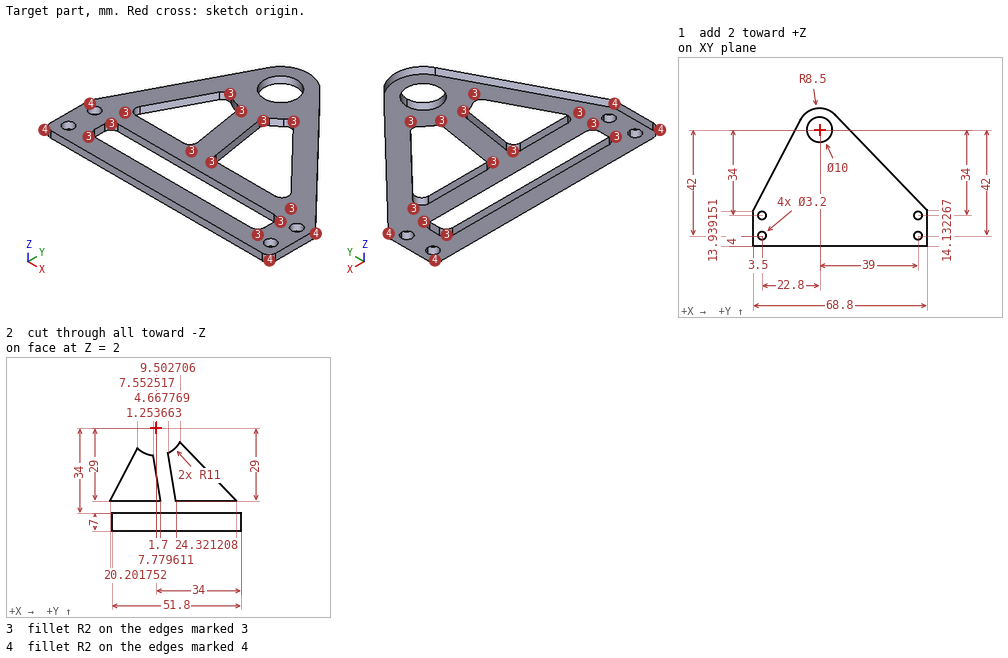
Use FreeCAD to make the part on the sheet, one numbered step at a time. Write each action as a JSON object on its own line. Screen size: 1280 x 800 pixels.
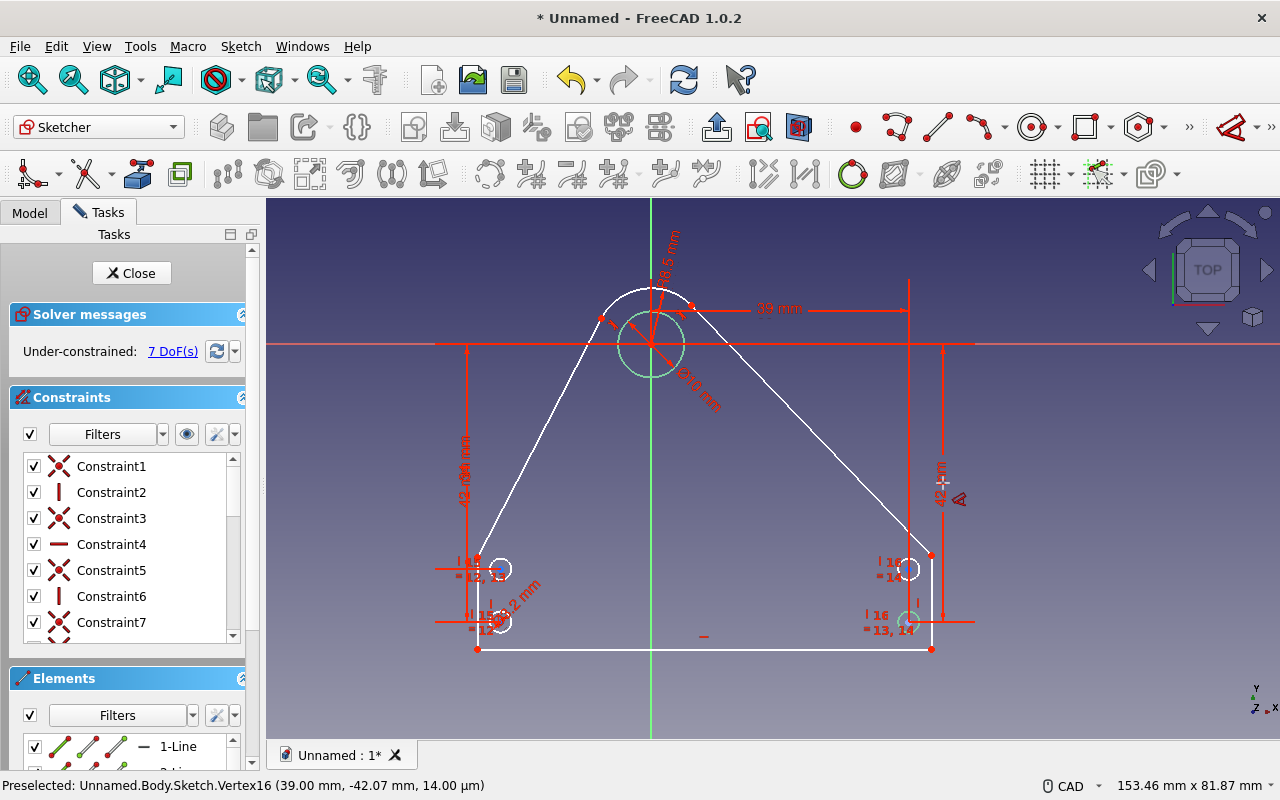
{"action": "left_click", "coordinate": [909, 569]}
{"action": "left_click", "coordinate": [943, 457]}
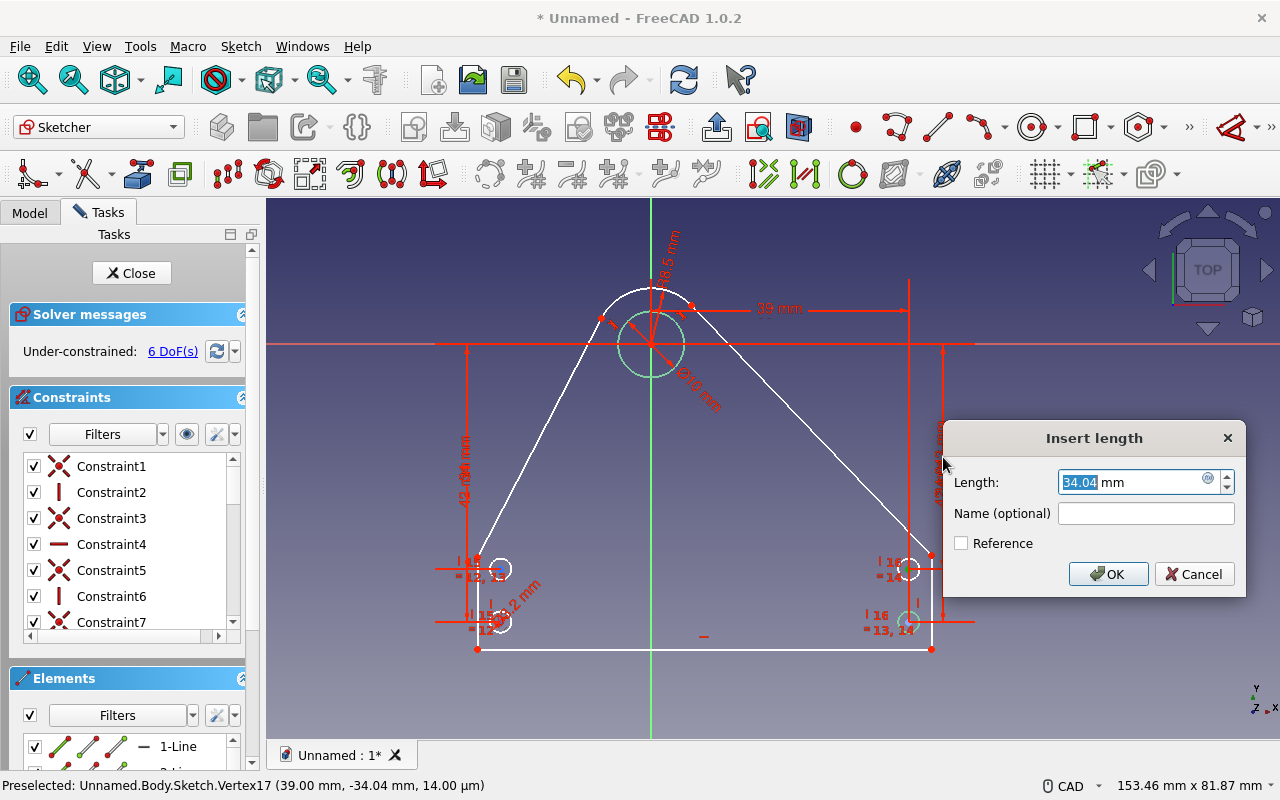
{"action": "type", "text": "34"}
{"action": "key", "text": "Return"}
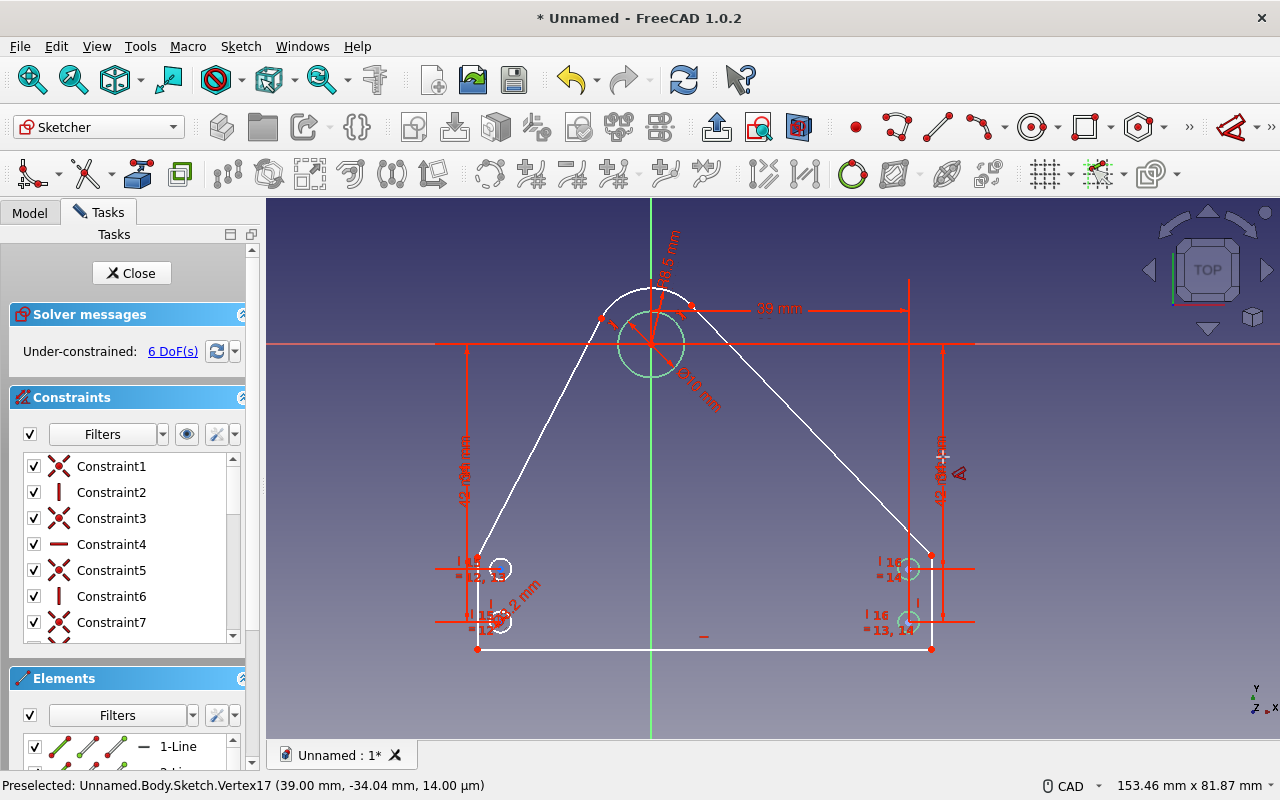
{"action": "scroll", "coordinate": [478, 650], "scroll_direction": "up", "scroll_amount": 3}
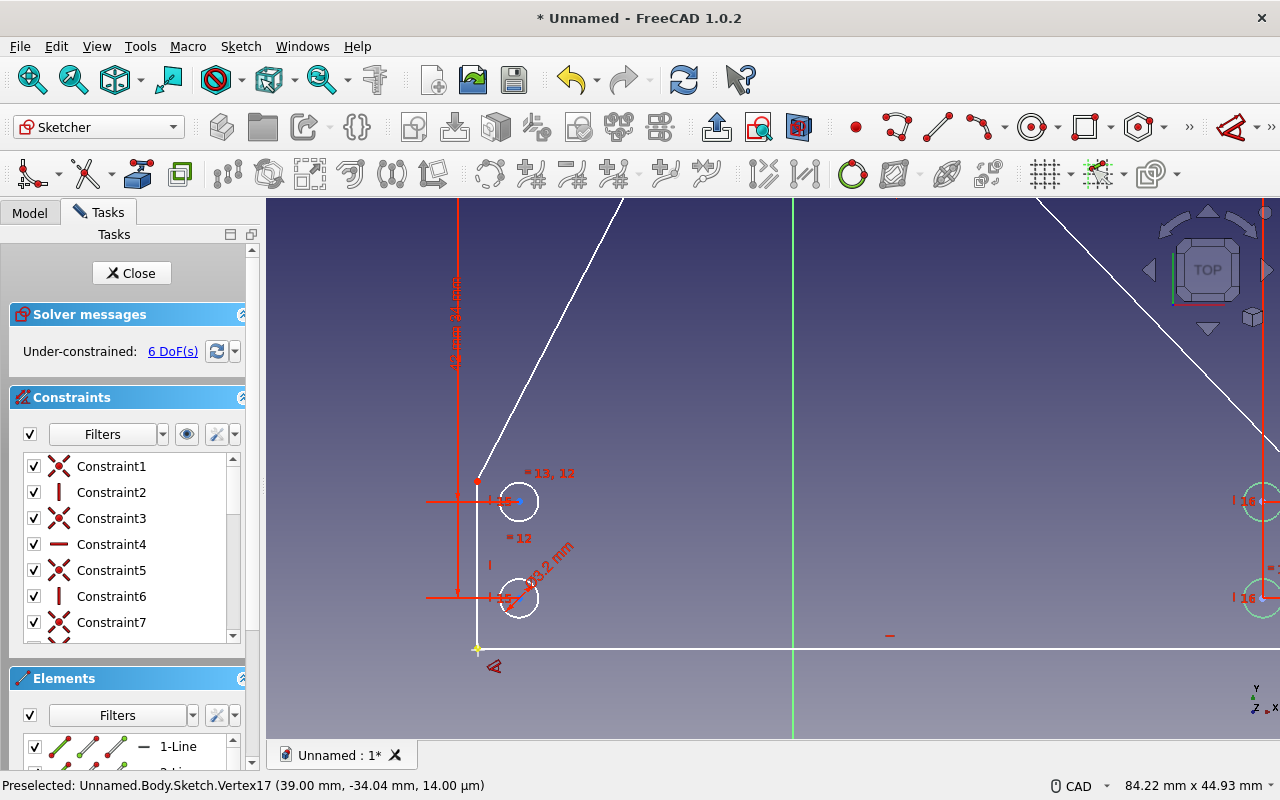
{"action": "left_click", "coordinate": [477, 649]}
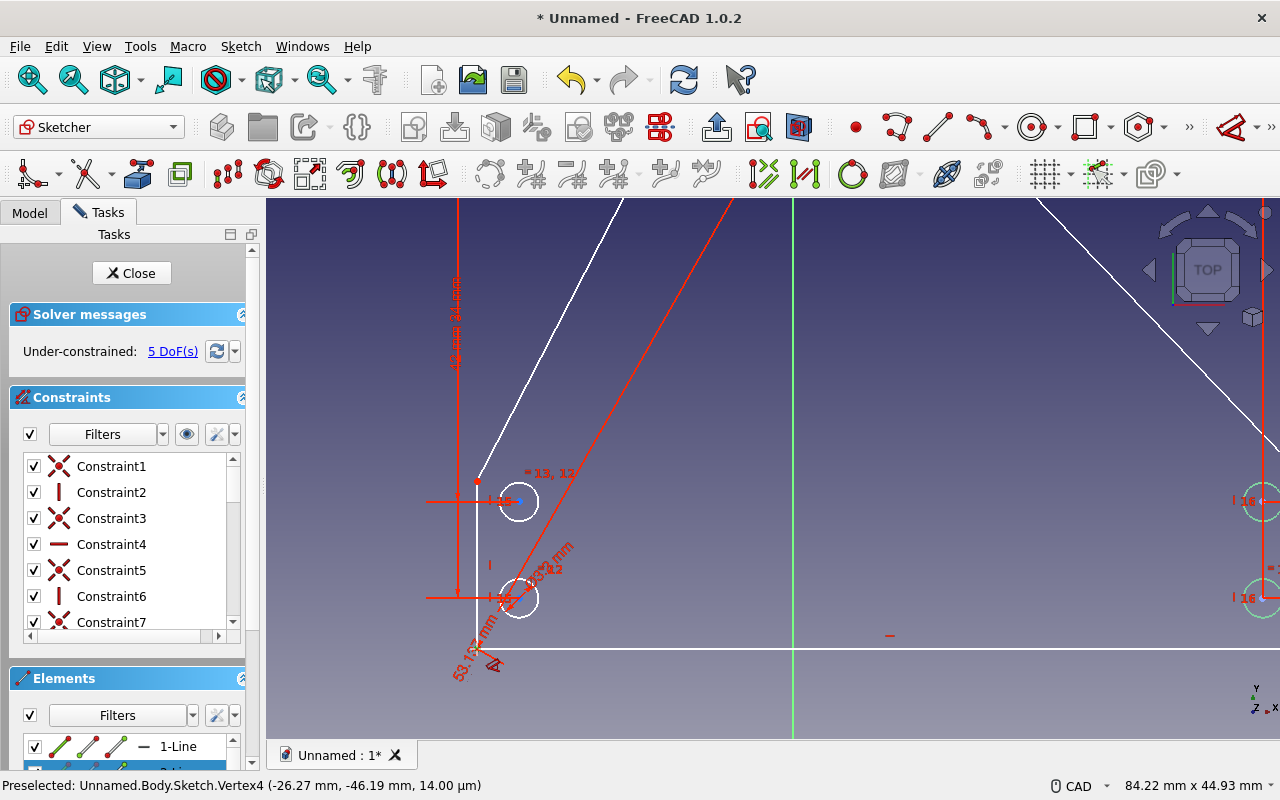
{"action": "left_click", "coordinate": [519, 598]}
{"action": "left_click", "coordinate": [443, 624]}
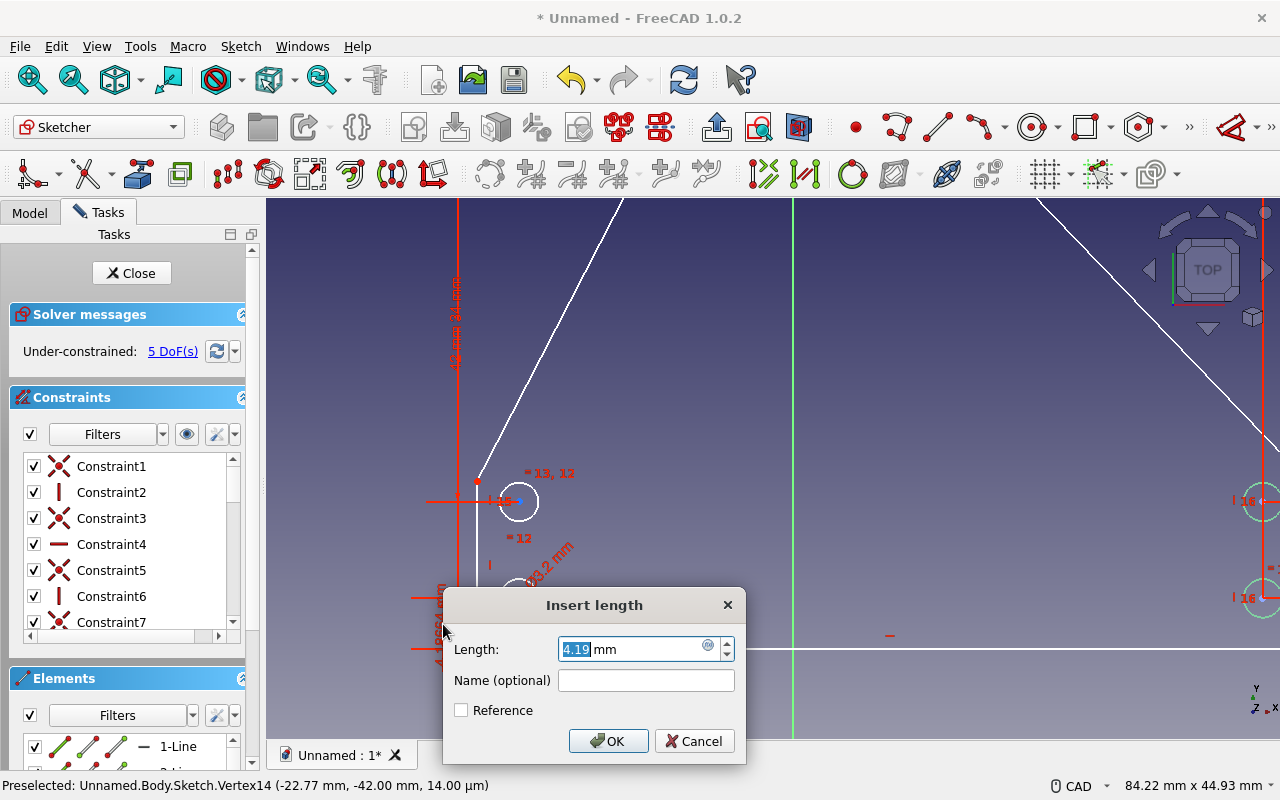
{"action": "type", "text": "4"}
{"action": "key", "text": "Return"}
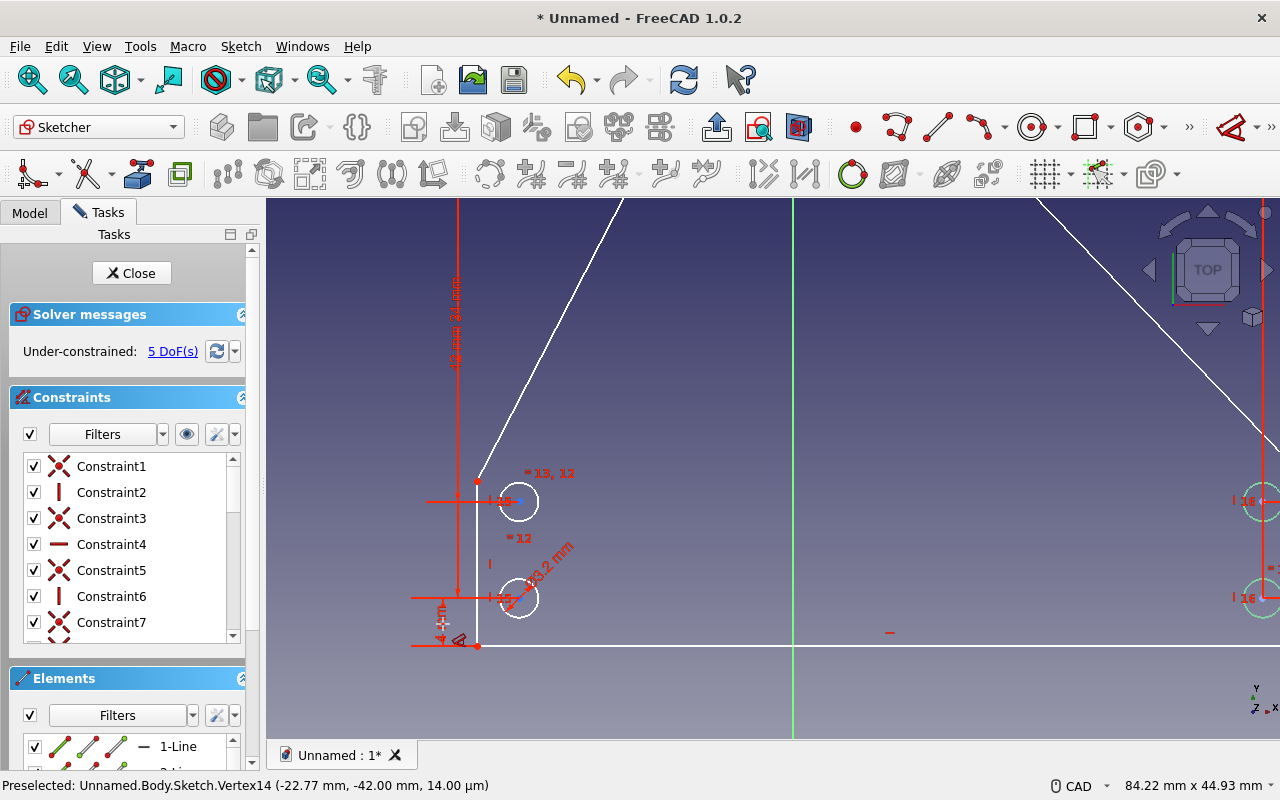
{"action": "left_click", "coordinate": [725, 646]}
{"action": "left_click", "coordinate": [649, 680]}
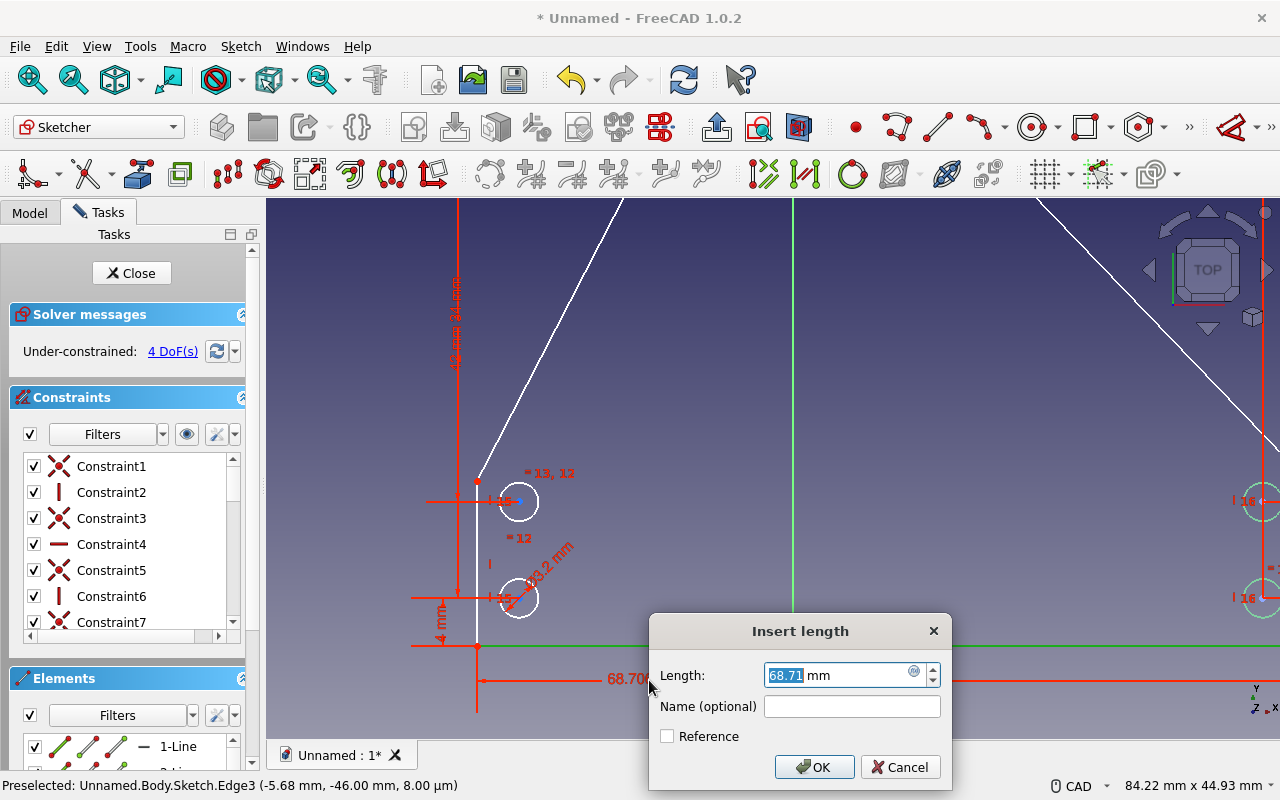
{"action": "type", "text": "68.8"}
{"action": "key", "text": "Return"}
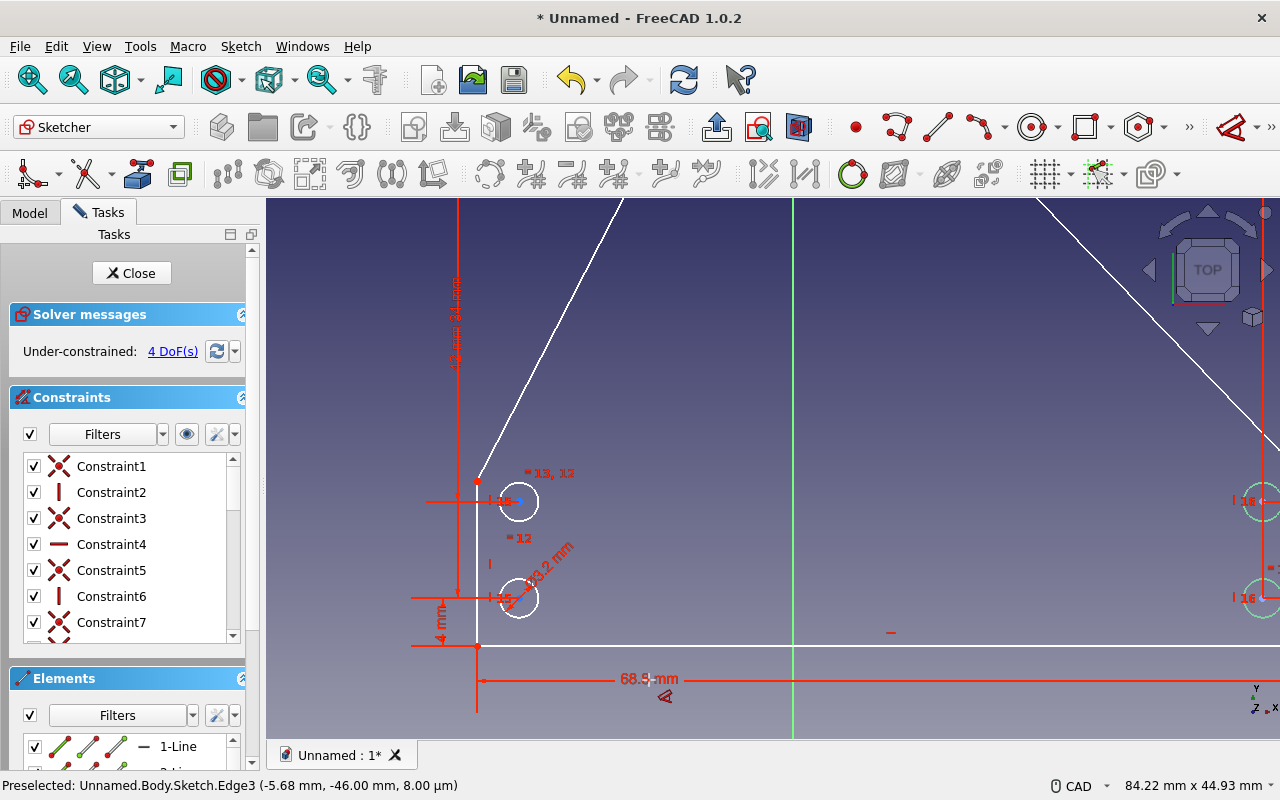
{"action": "left_click", "coordinate": [519, 598]}
{"action": "left_click", "coordinate": [656, 632]}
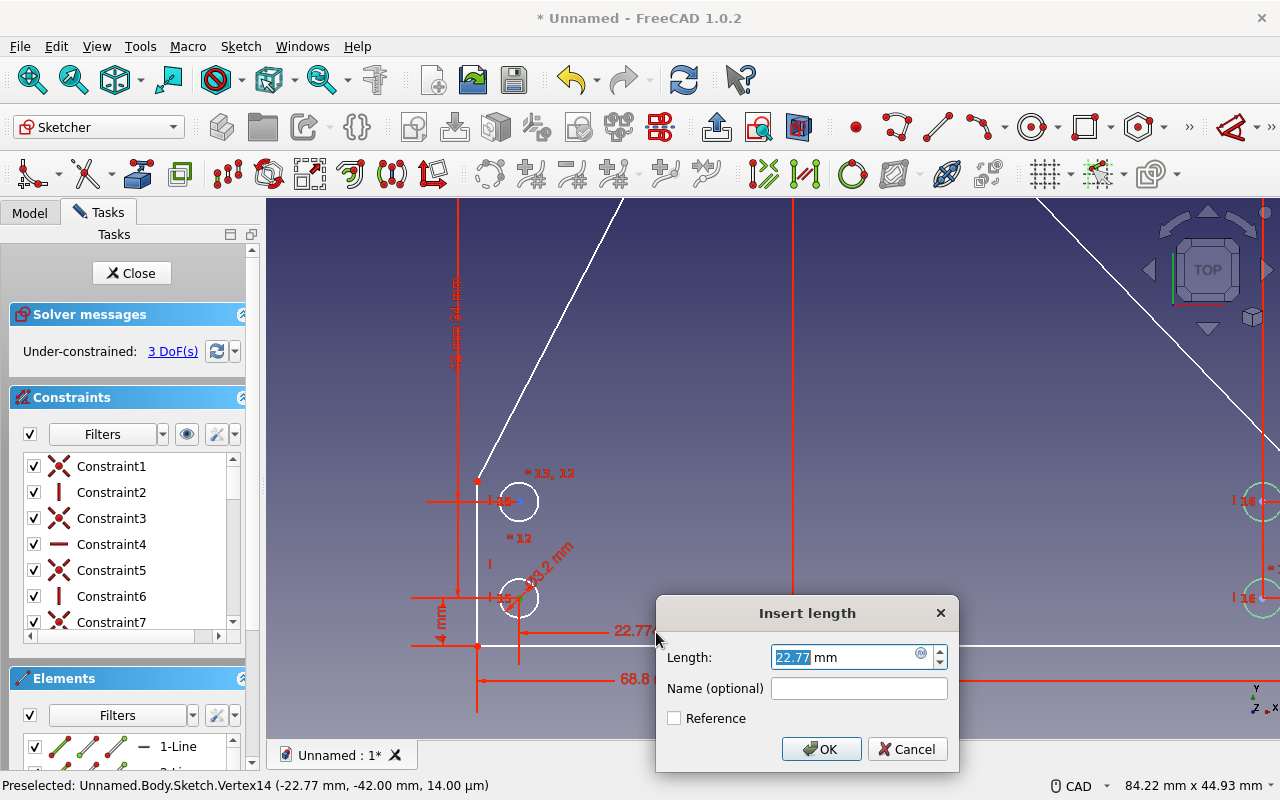
{"action": "type", "text": "22.8"}
{"action": "key", "text": "Return"}